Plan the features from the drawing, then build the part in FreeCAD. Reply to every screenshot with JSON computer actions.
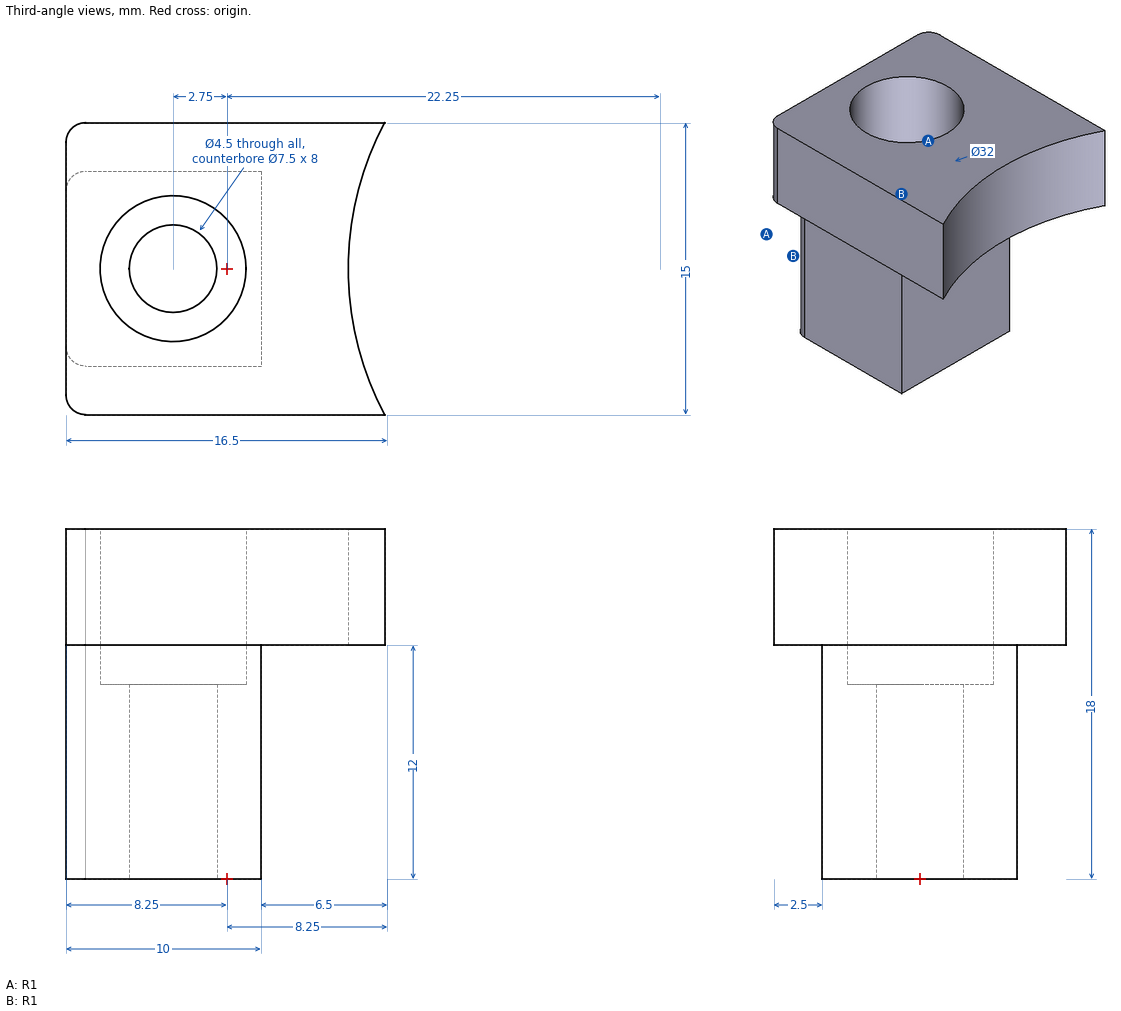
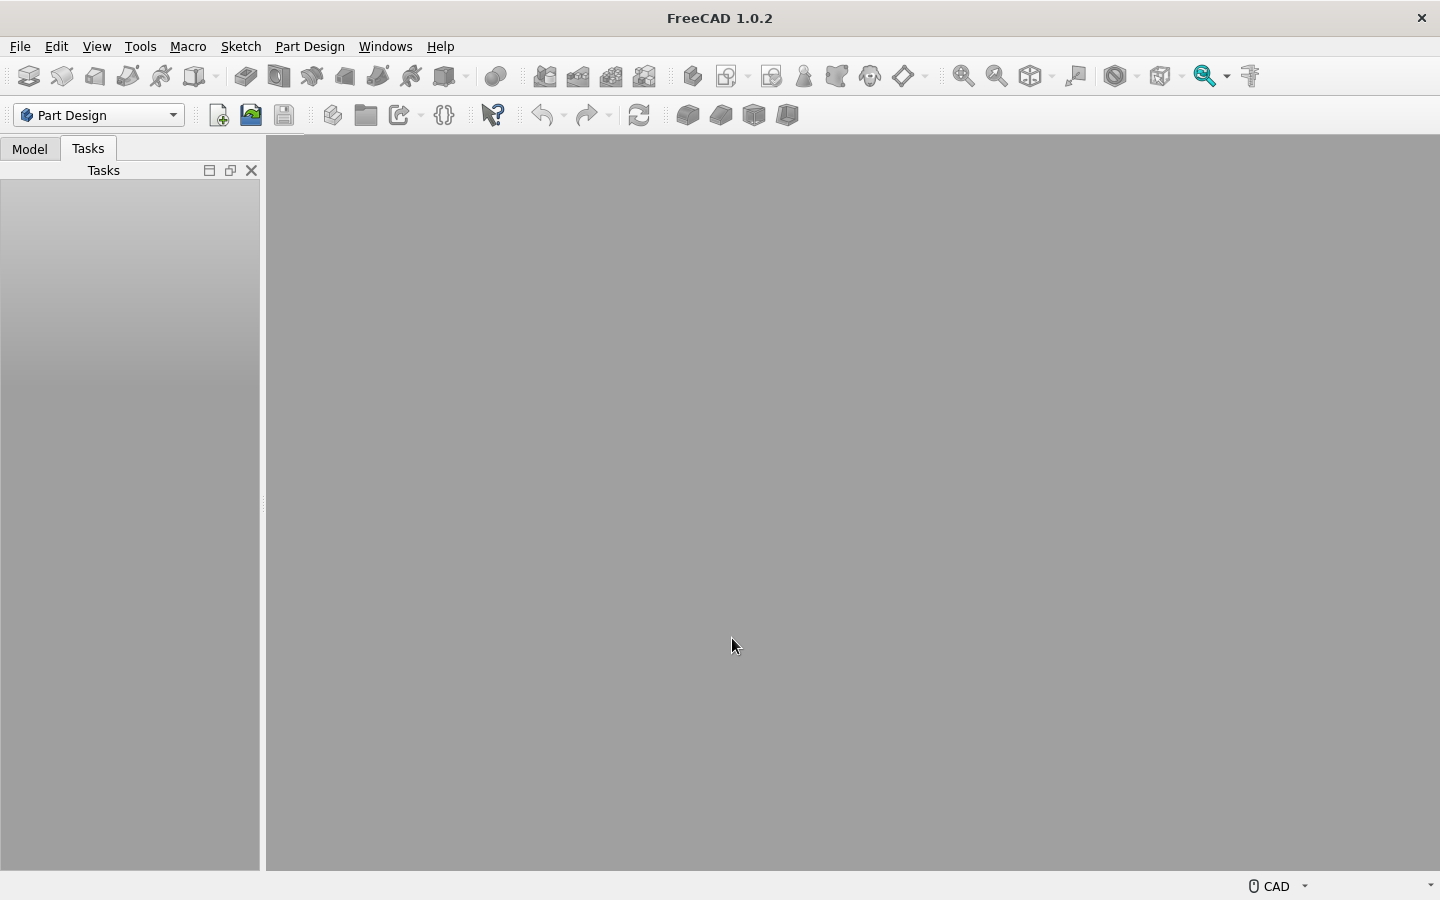
{"action": "key", "text": "ctrl+n"}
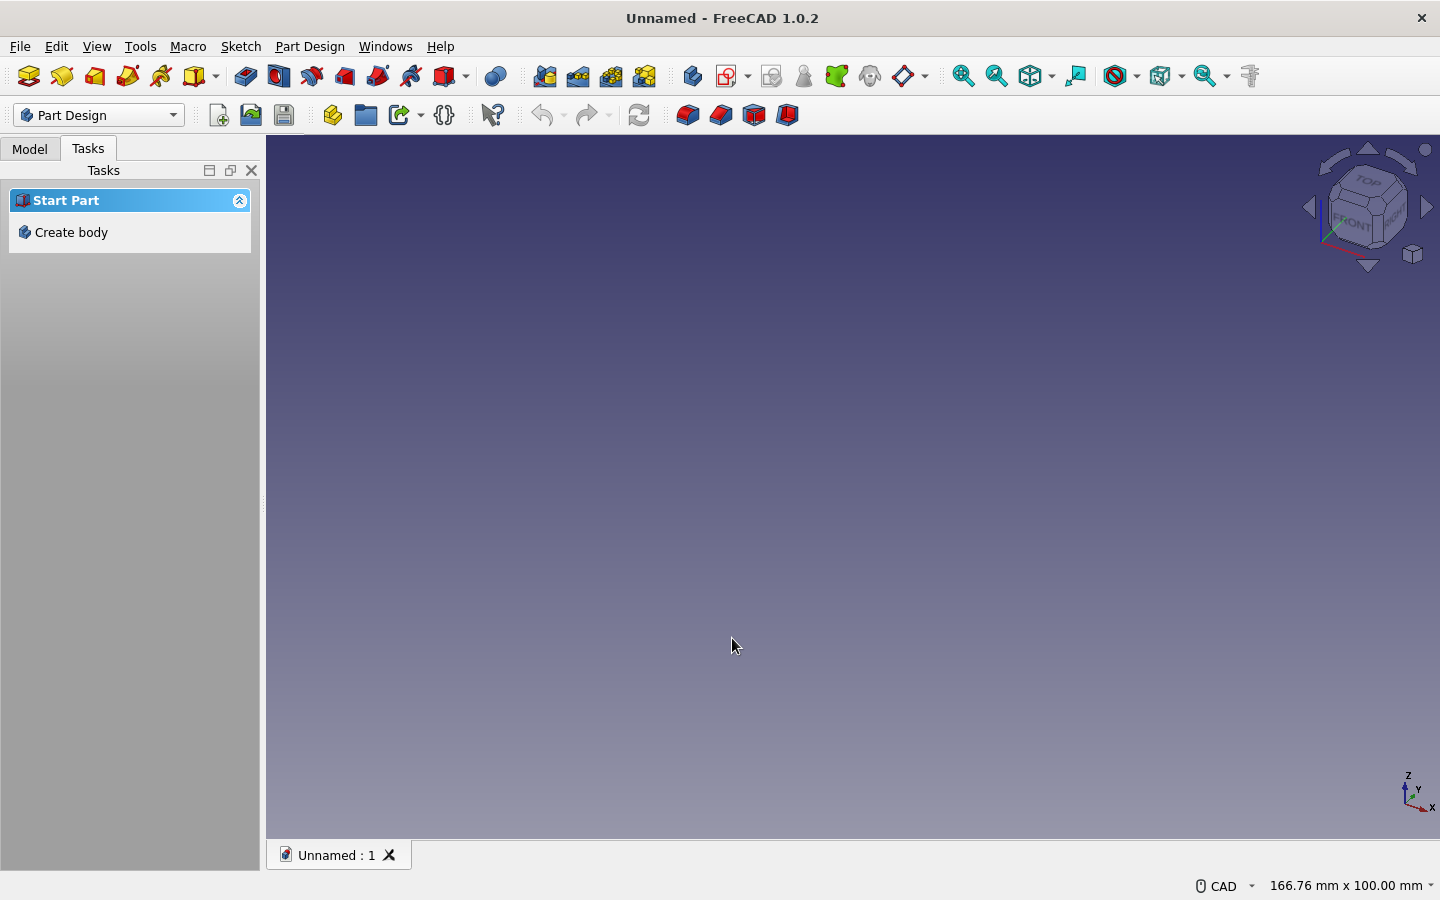
{"action": "left_click", "coordinate": [726, 76]}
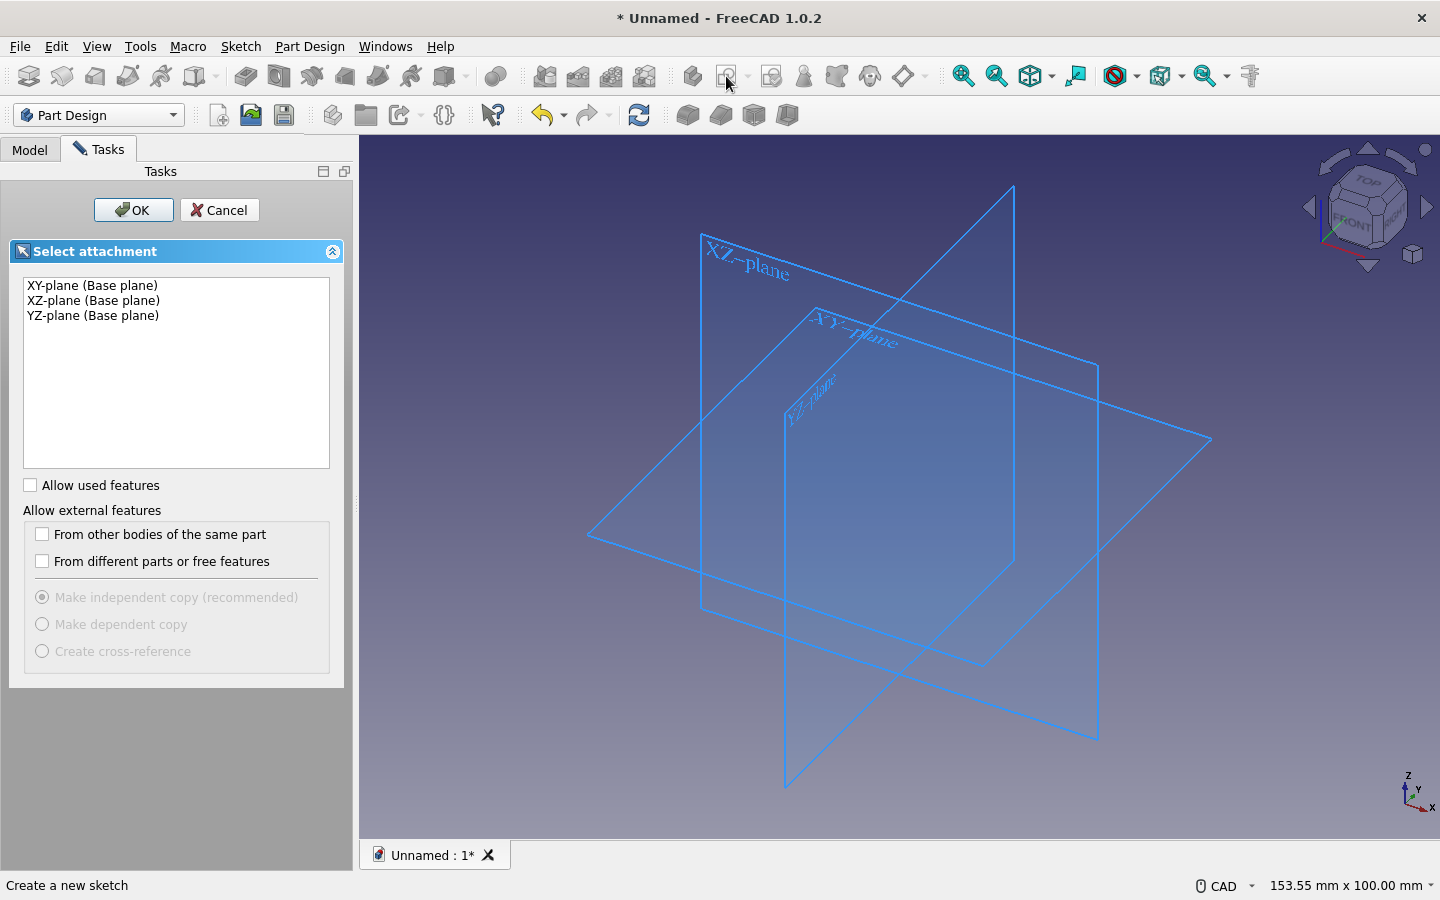
{"action": "left_click", "coordinate": [84, 286]}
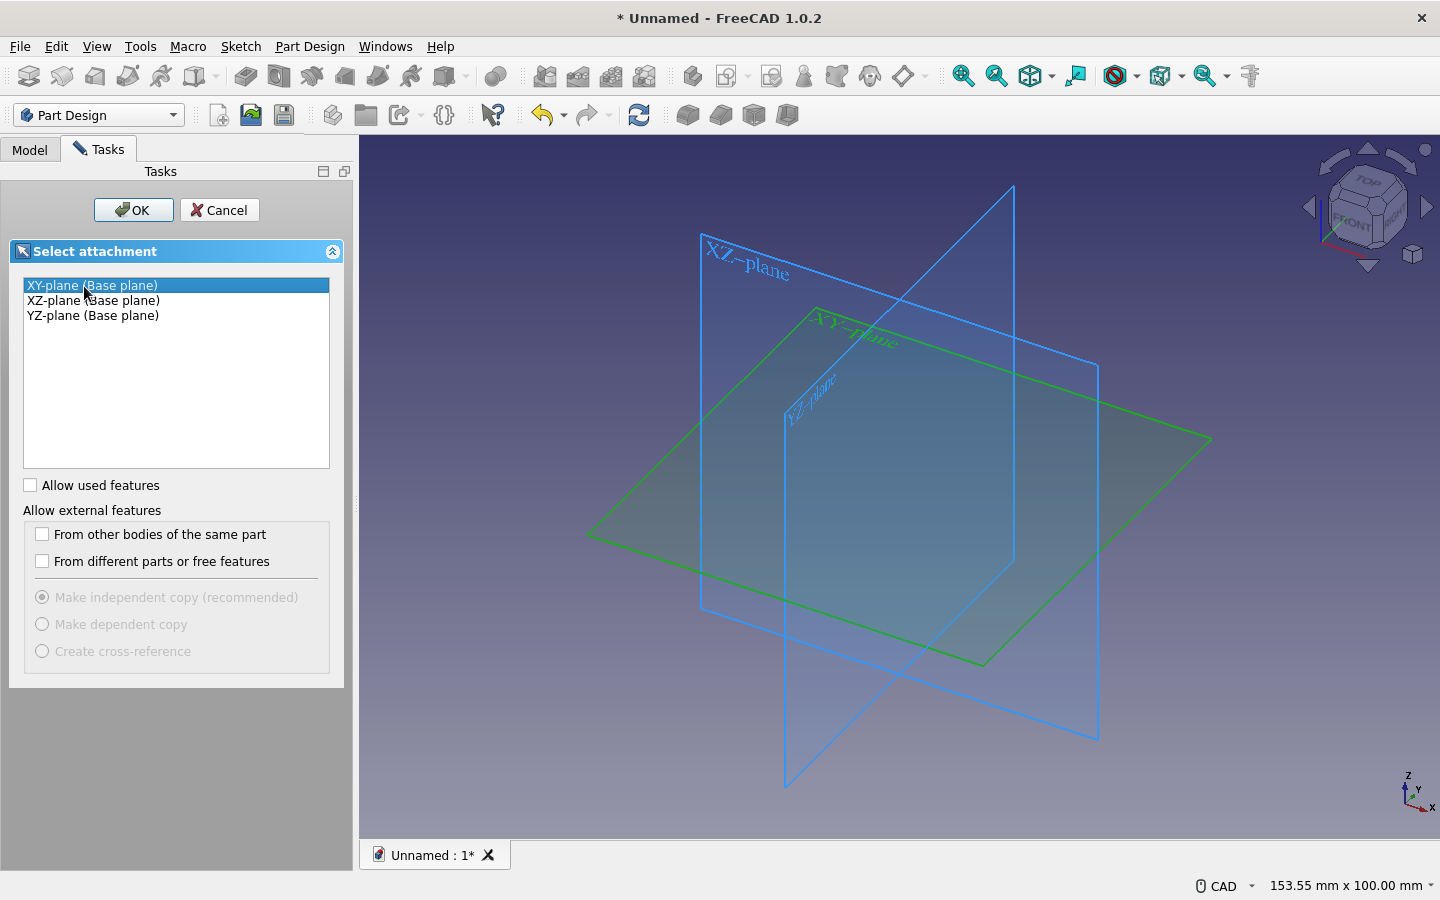
{"action": "left_click", "coordinate": [134, 210]}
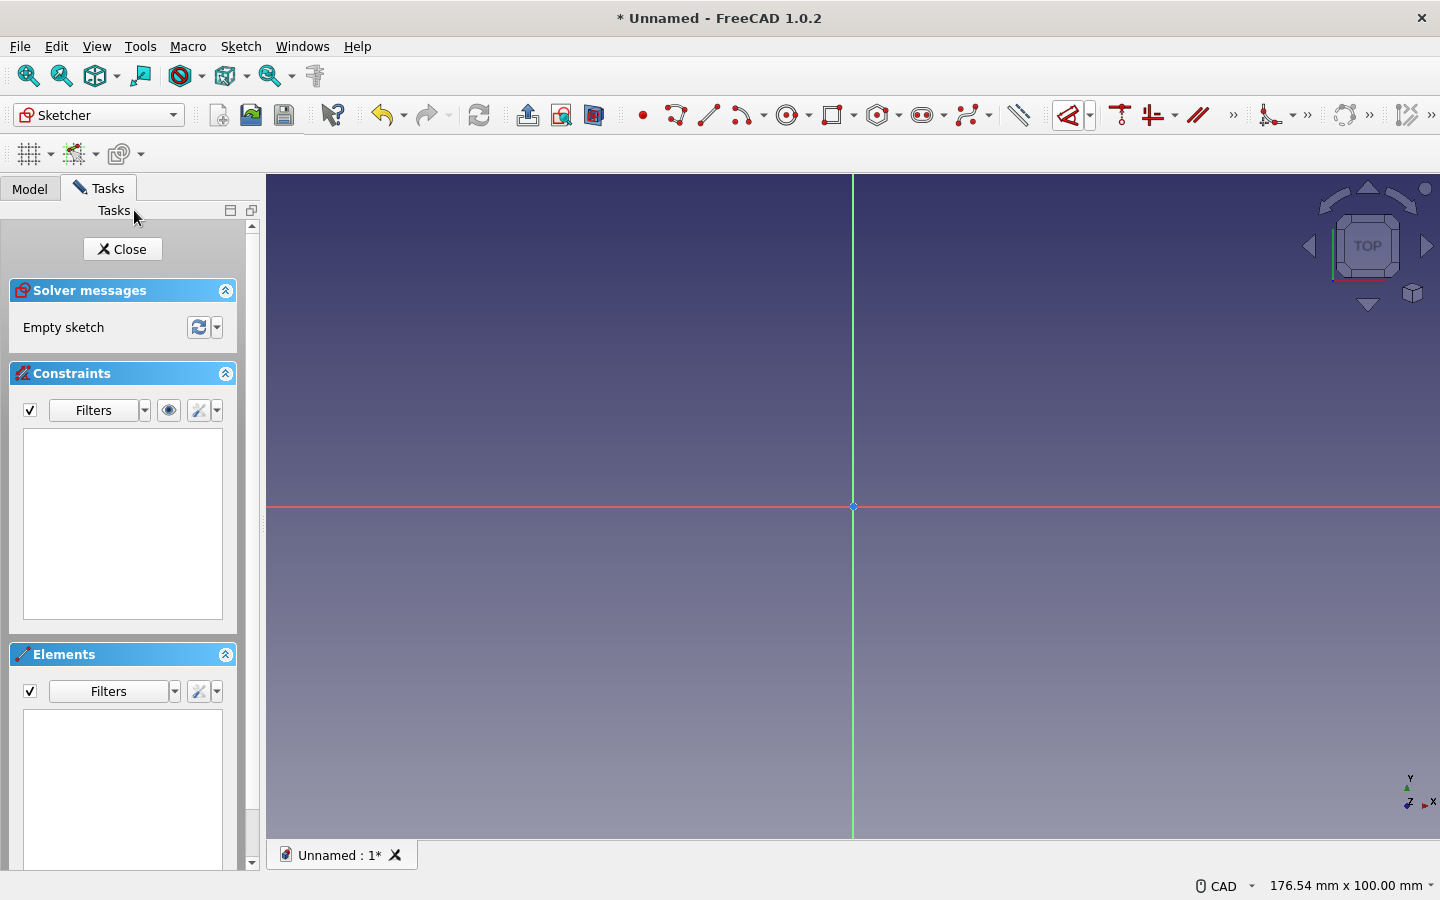
{"action": "scroll", "coordinate": [875, 507], "scroll_direction": "up", "scroll_amount": 7}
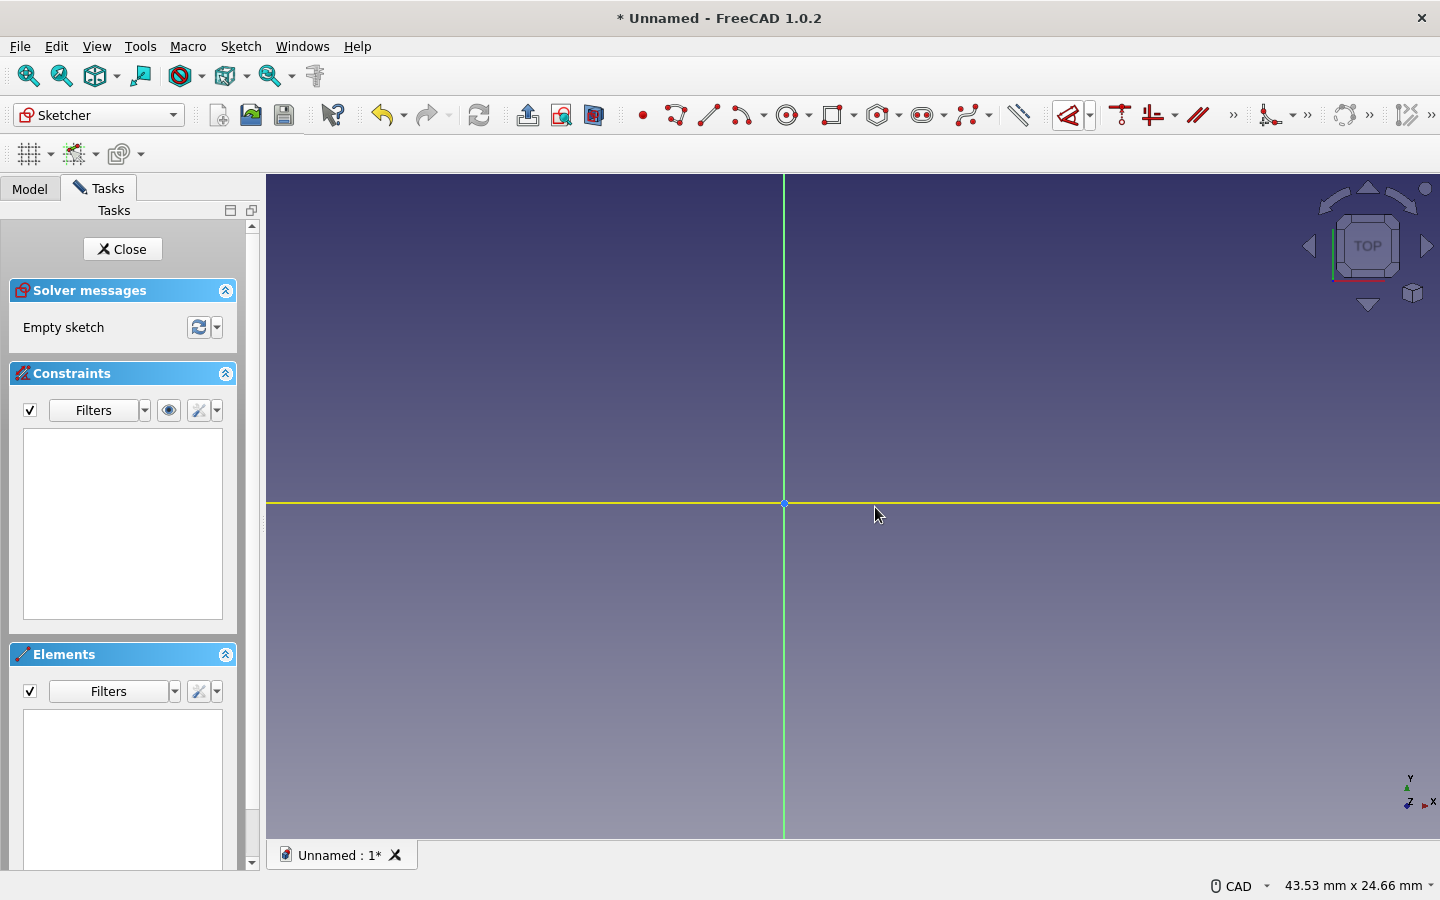
{"action": "key", "text": "g v"}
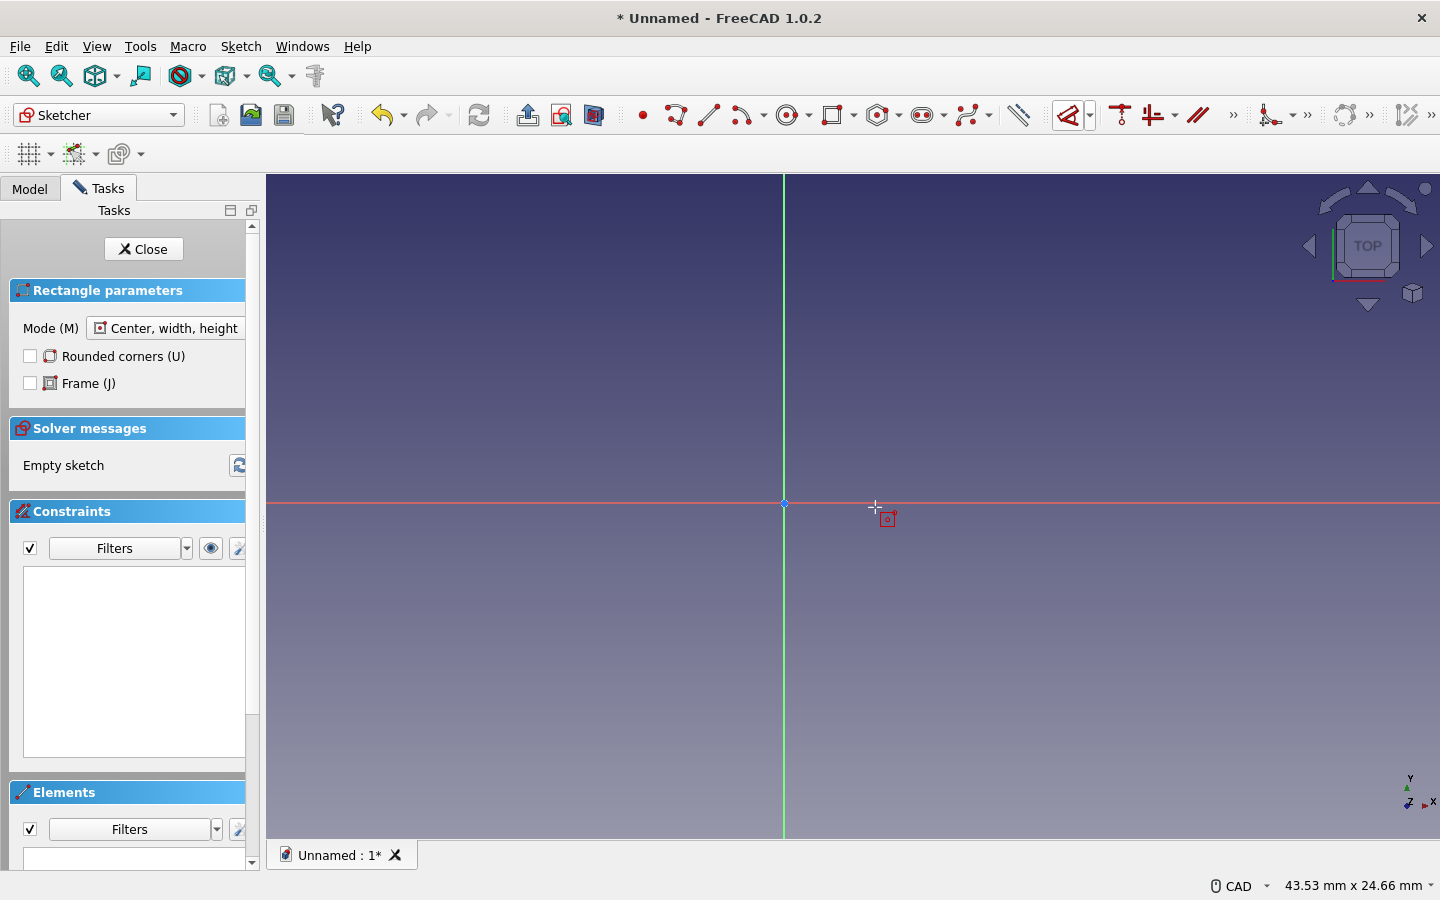
{"action": "left_click", "coordinate": [784, 503]}
{"action": "left_click", "coordinate": [1007, 301]}
{"action": "key", "text": "Escape"}